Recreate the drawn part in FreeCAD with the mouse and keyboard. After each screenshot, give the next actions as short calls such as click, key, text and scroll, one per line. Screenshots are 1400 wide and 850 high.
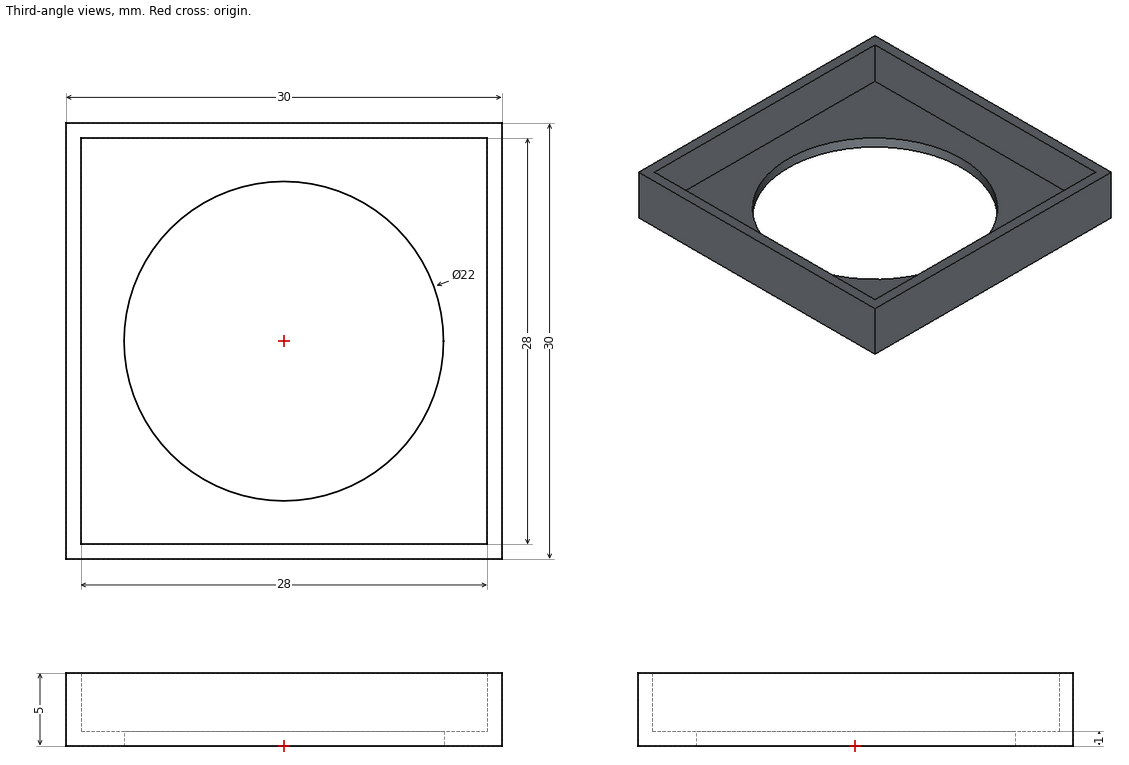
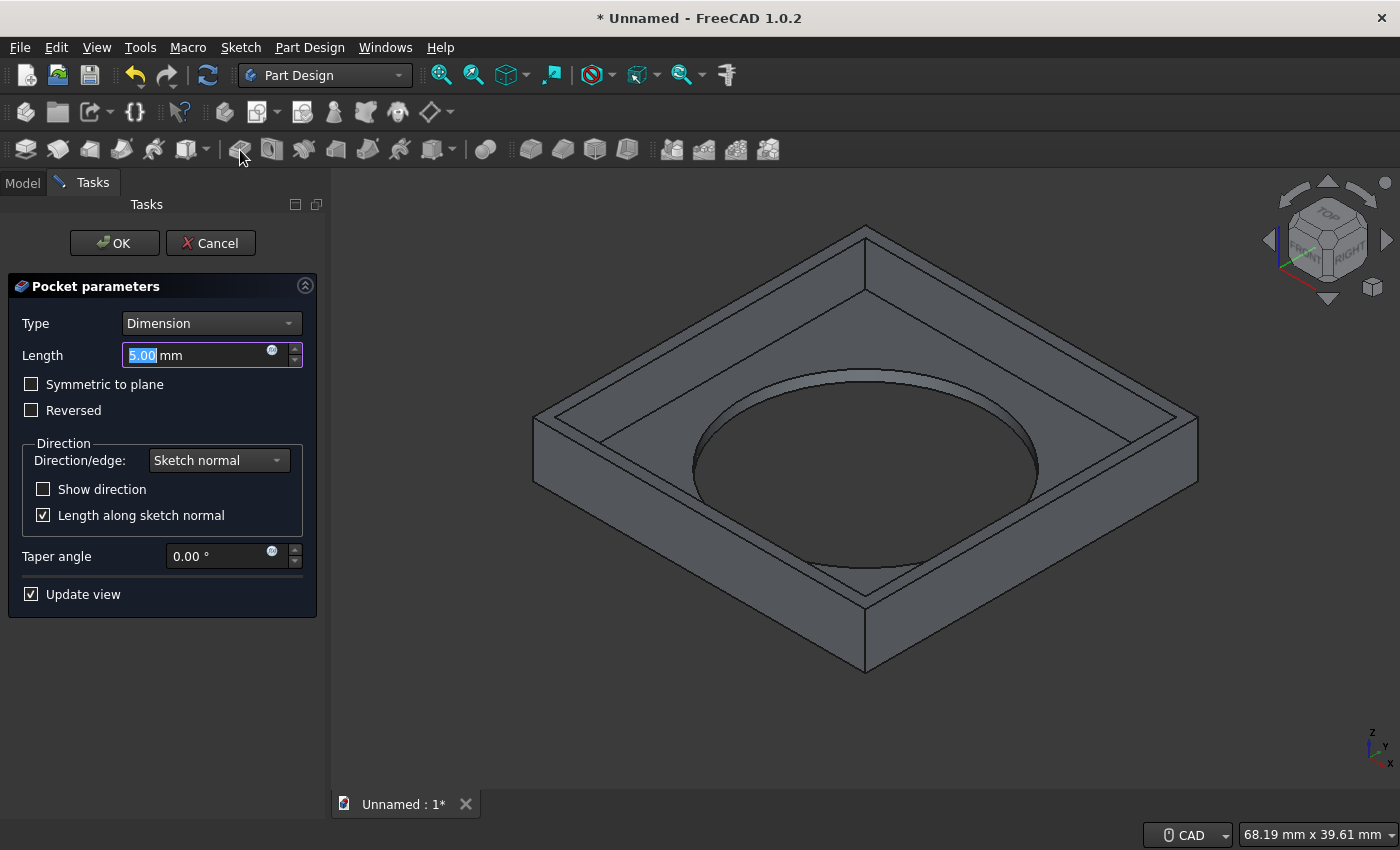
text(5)
key(Tab)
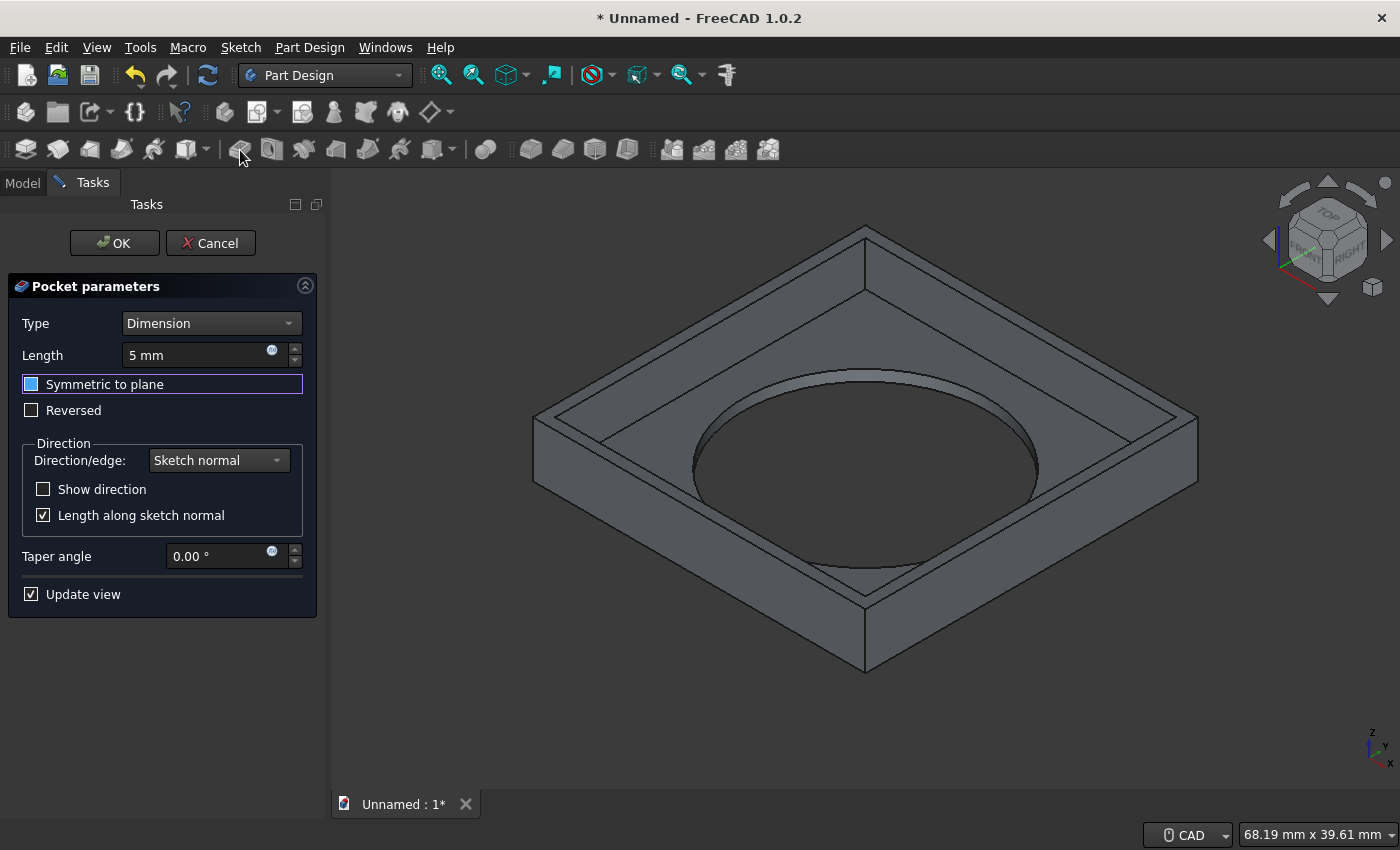
click(115, 243)